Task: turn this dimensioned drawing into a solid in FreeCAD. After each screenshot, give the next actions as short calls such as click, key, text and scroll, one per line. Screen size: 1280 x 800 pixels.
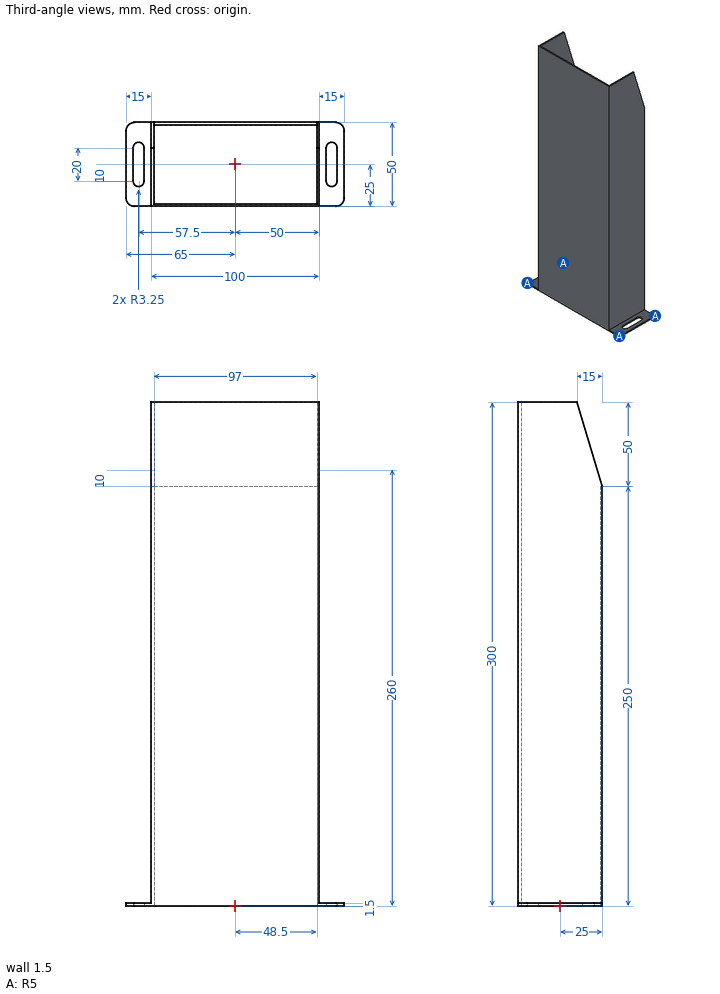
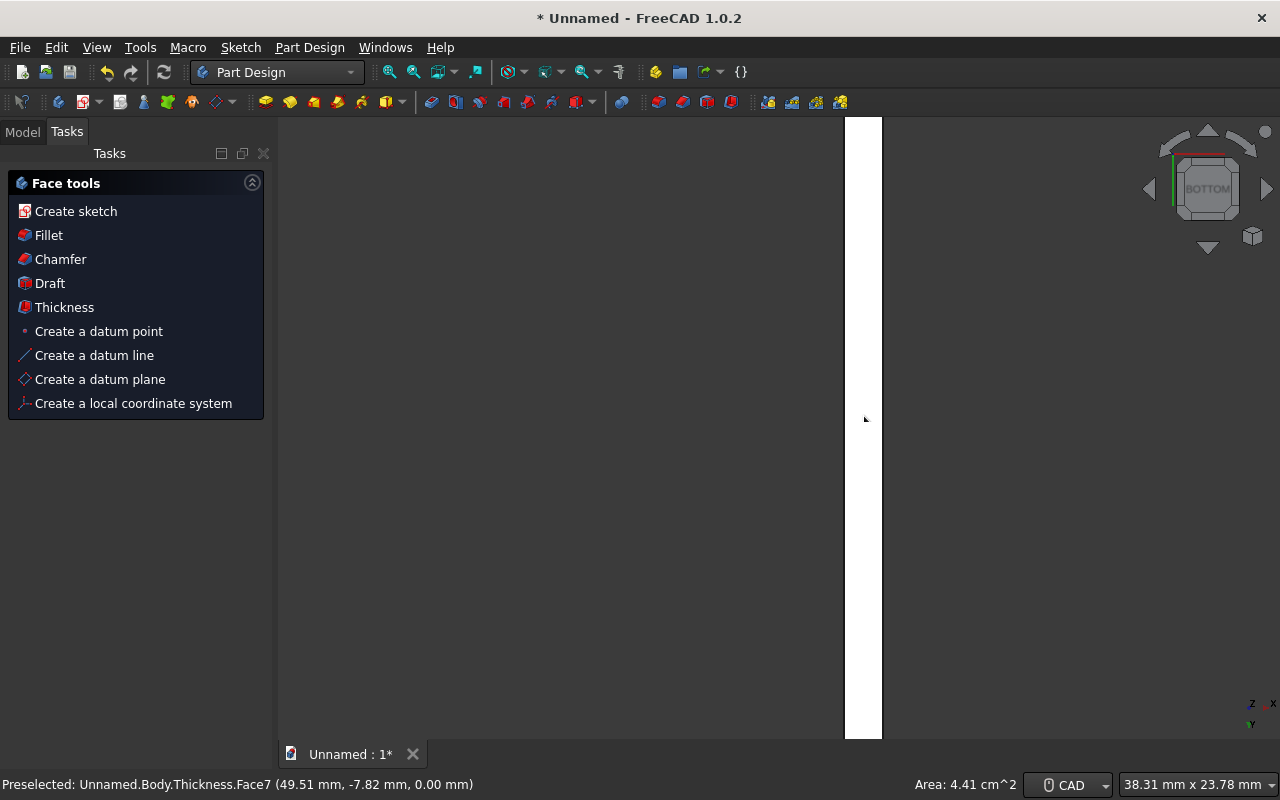
click(84, 102)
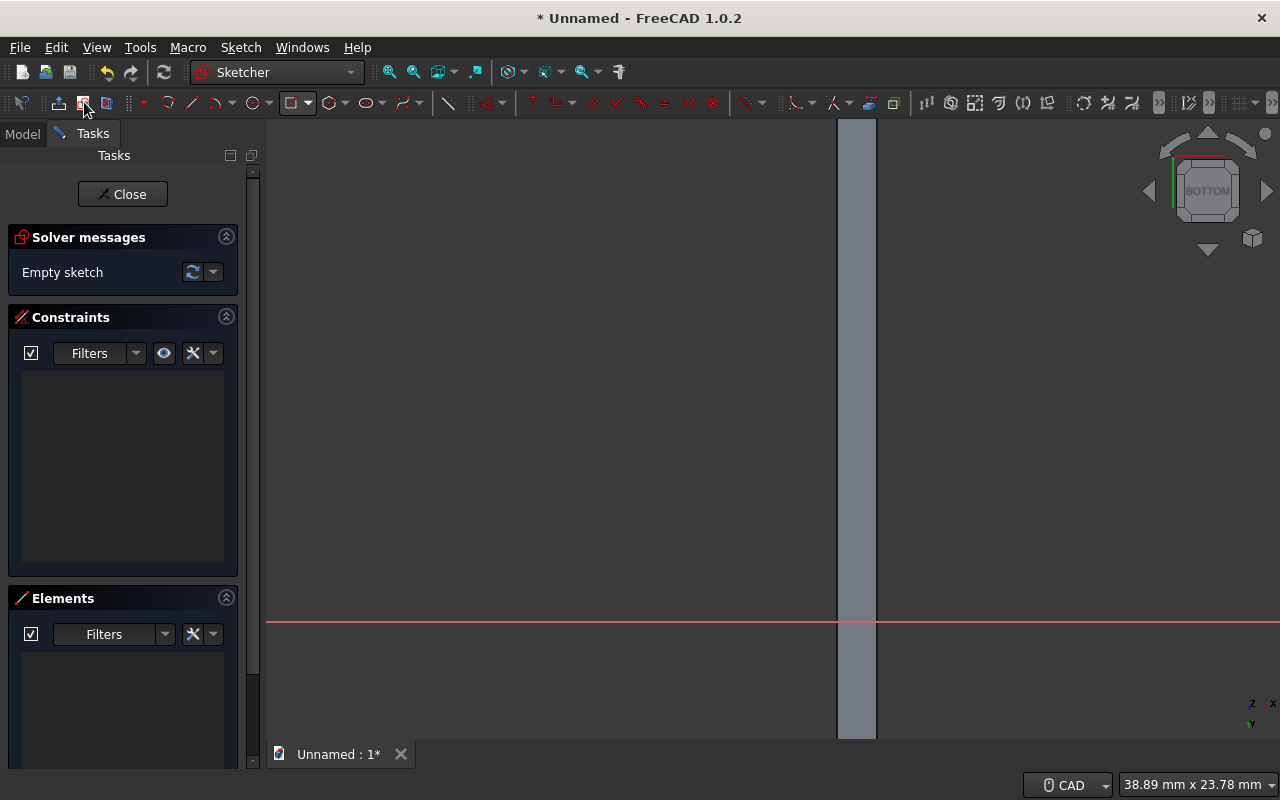
scroll(929, 391, down, 9)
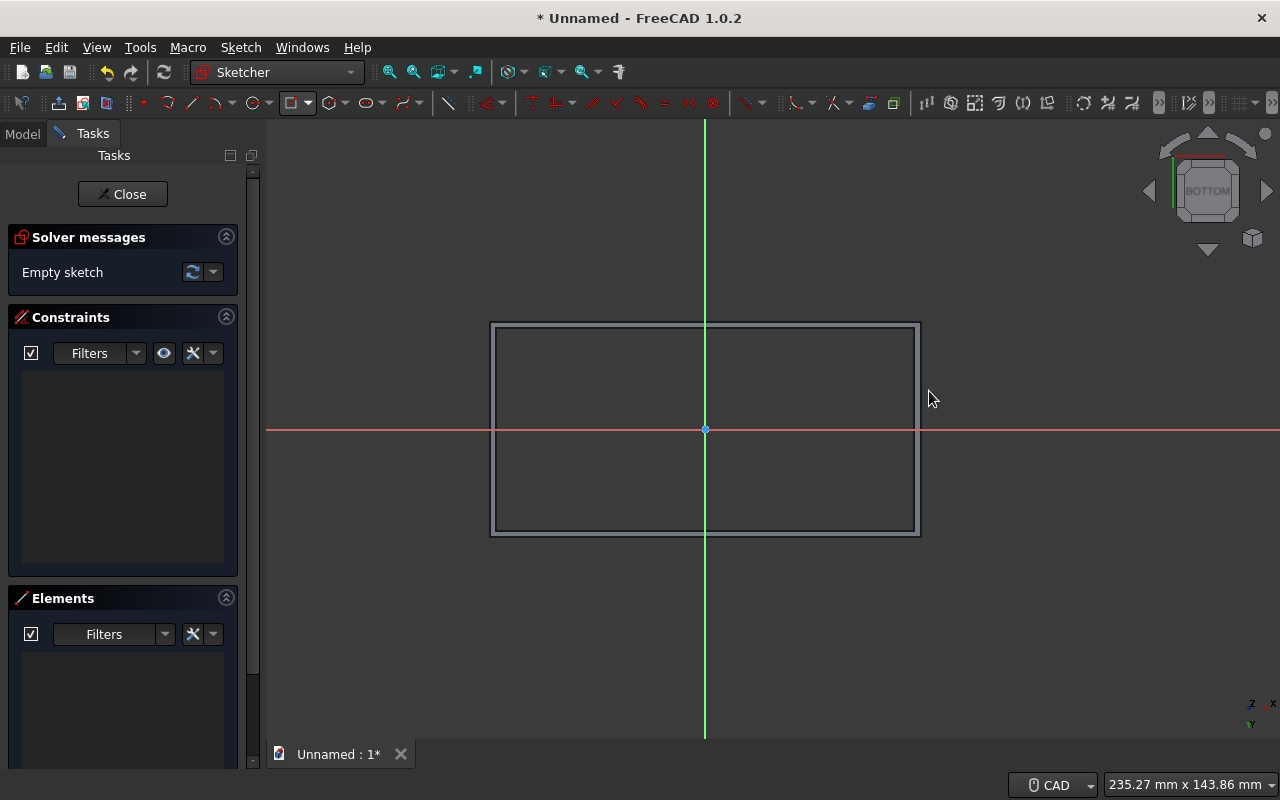
click(310, 104)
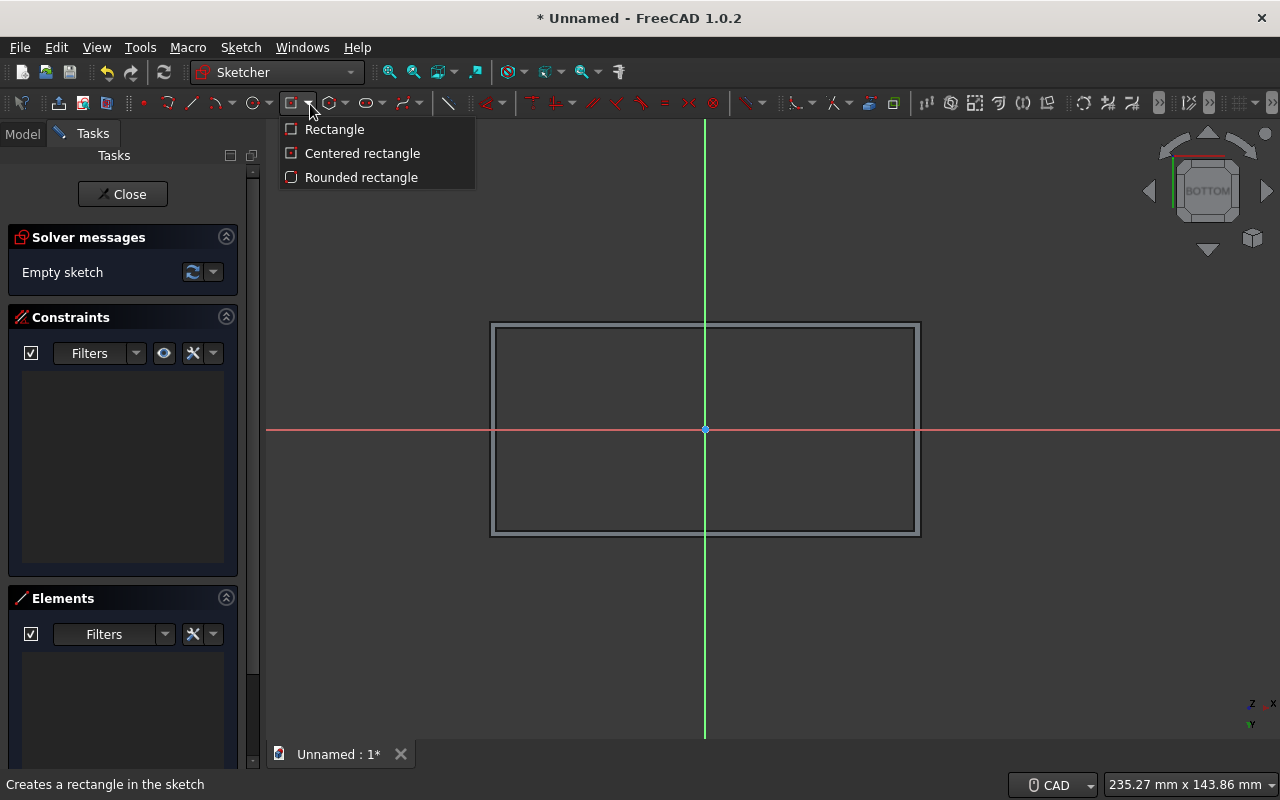
click(378, 129)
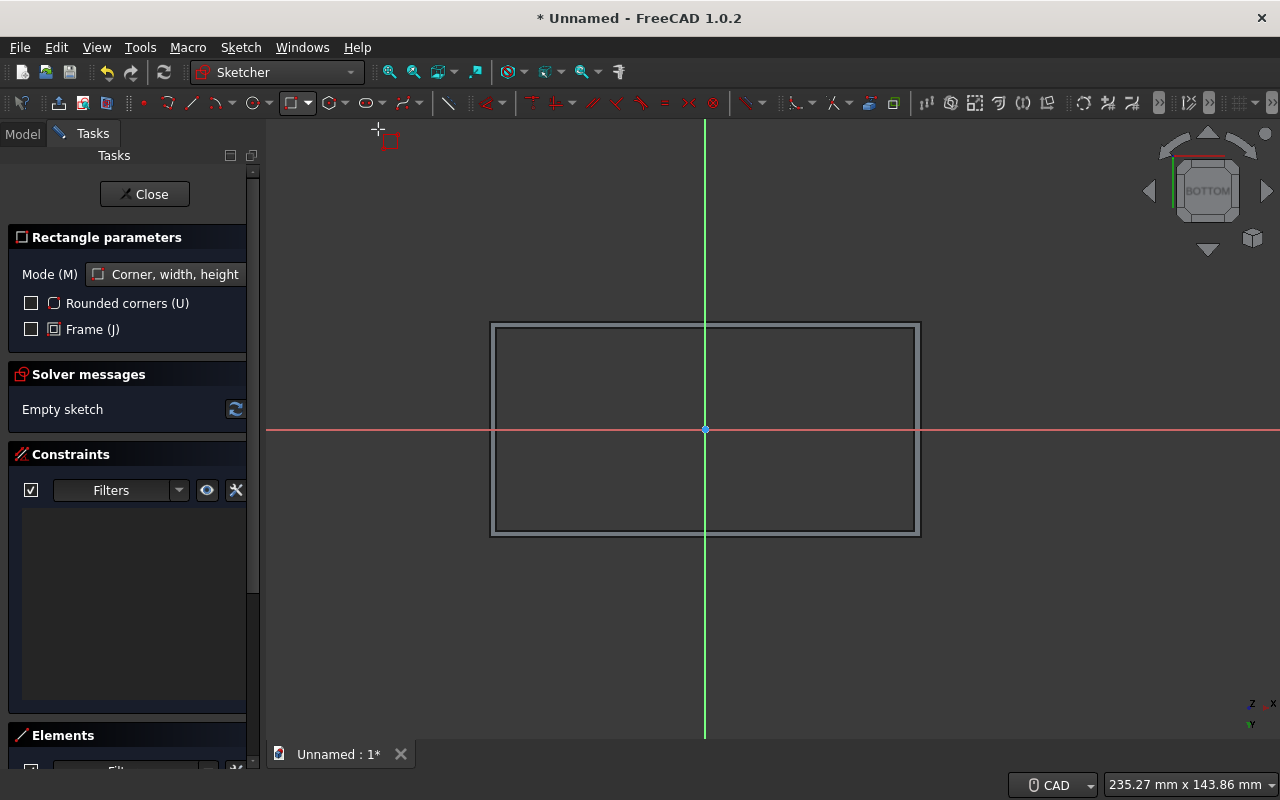
click(921, 322)
move(986, 537)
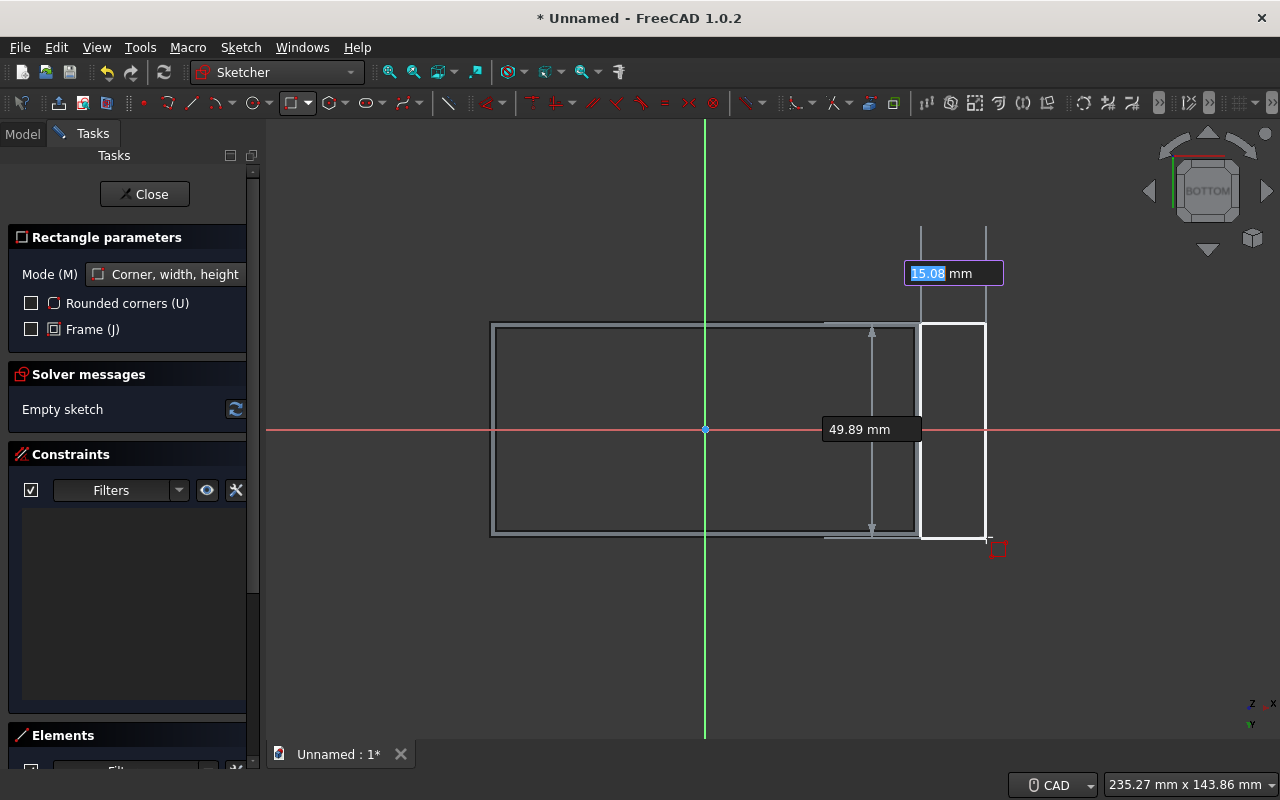
text(15)
key(Tab)
text(50)
key(Return)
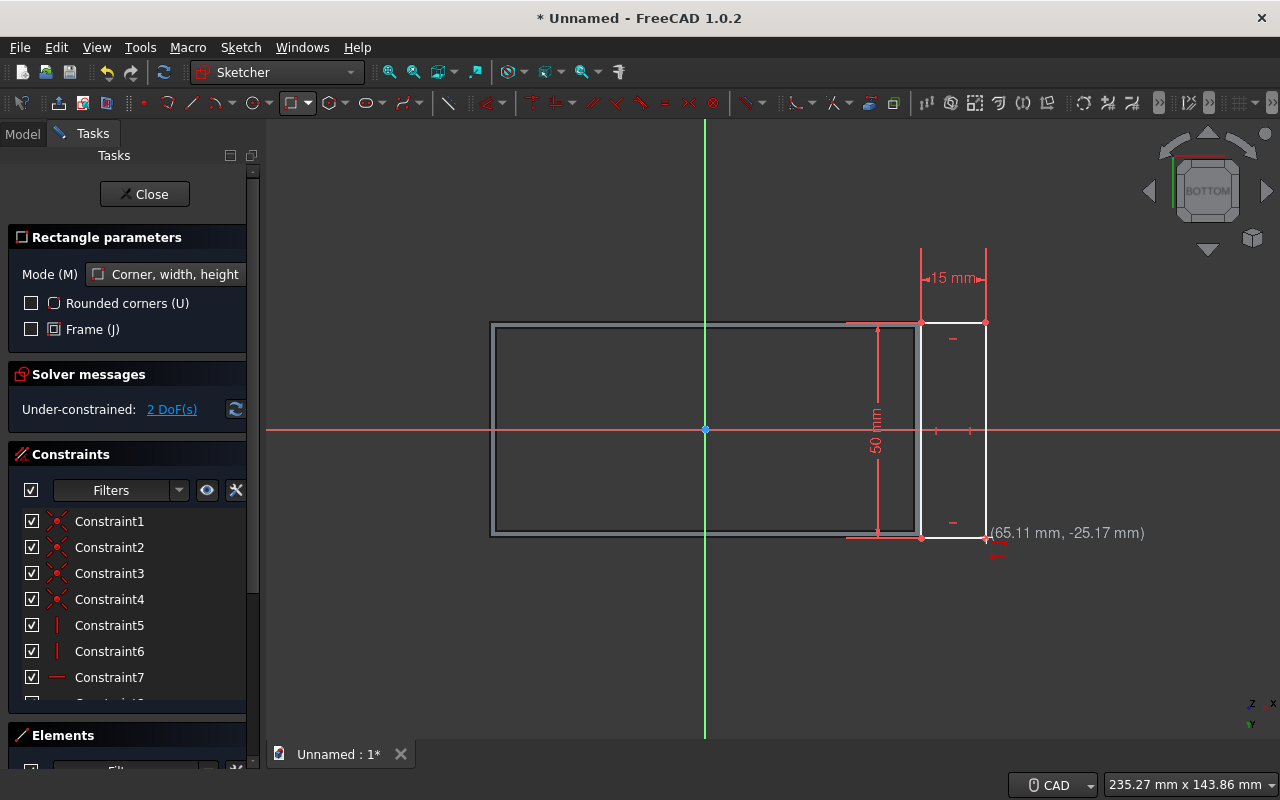
click(425, 322)
move(490, 537)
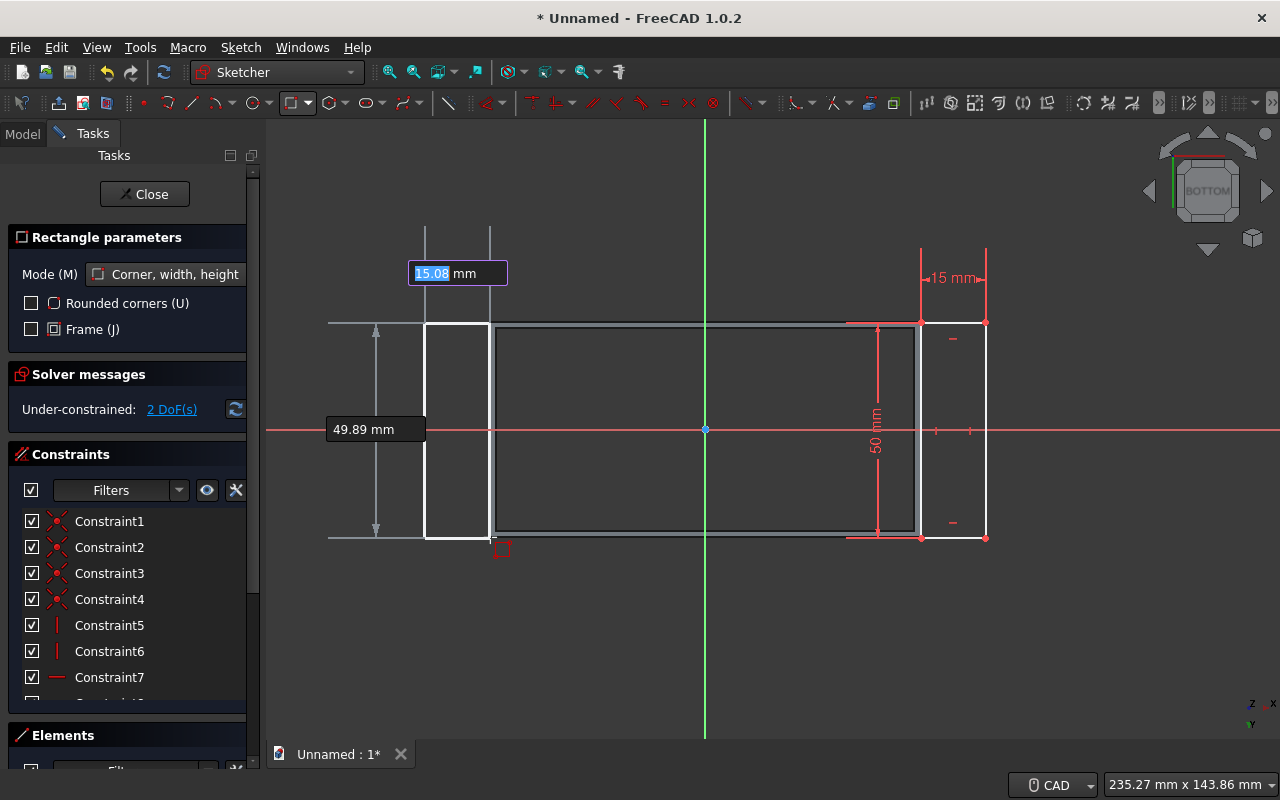
text(15)
key(Tab)
text(50)
key(Return)
key(Escape)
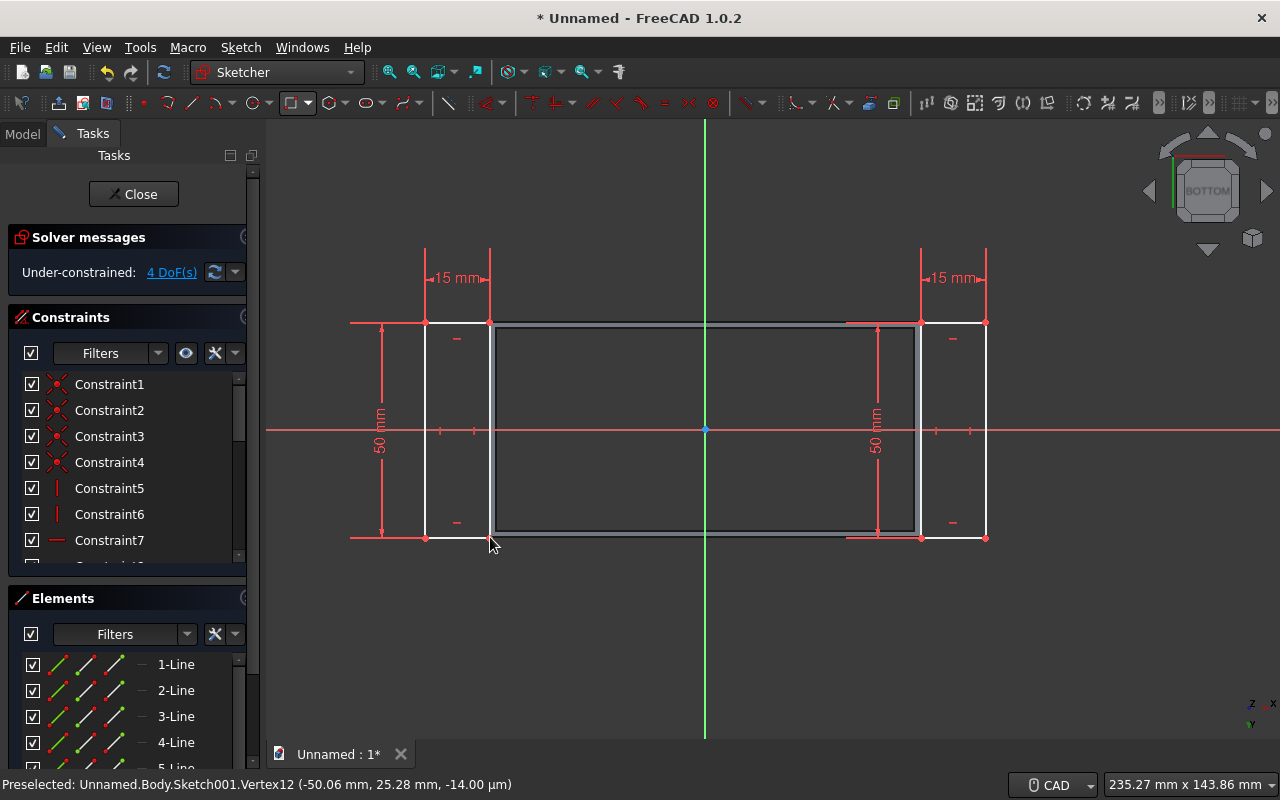
click(486, 104)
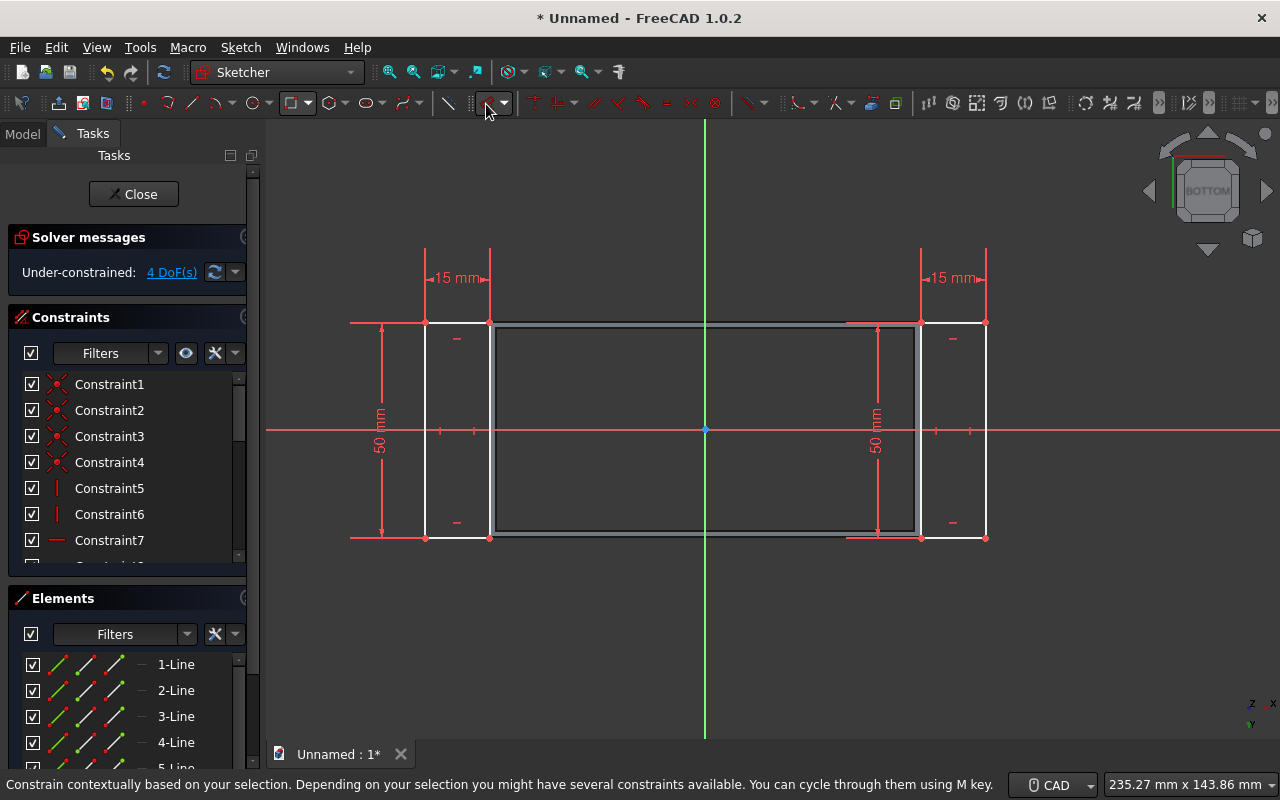
click(921, 323)
click(813, 289)